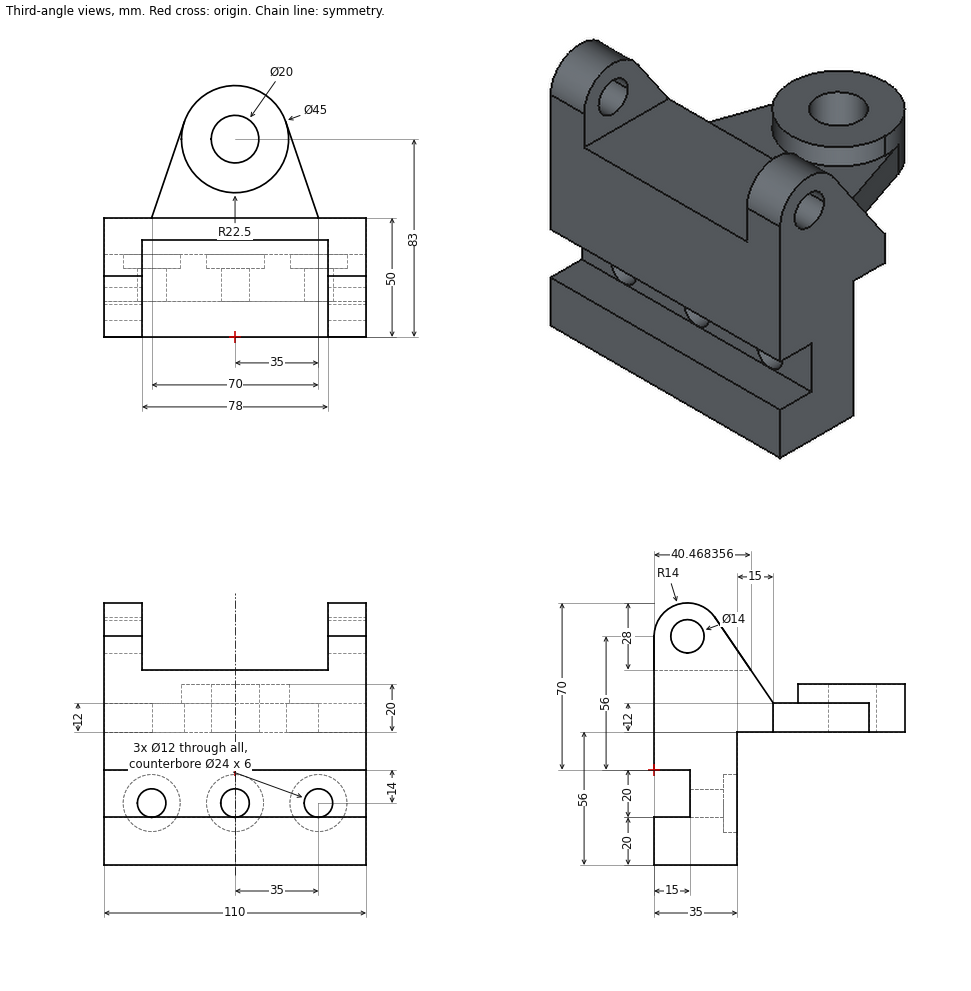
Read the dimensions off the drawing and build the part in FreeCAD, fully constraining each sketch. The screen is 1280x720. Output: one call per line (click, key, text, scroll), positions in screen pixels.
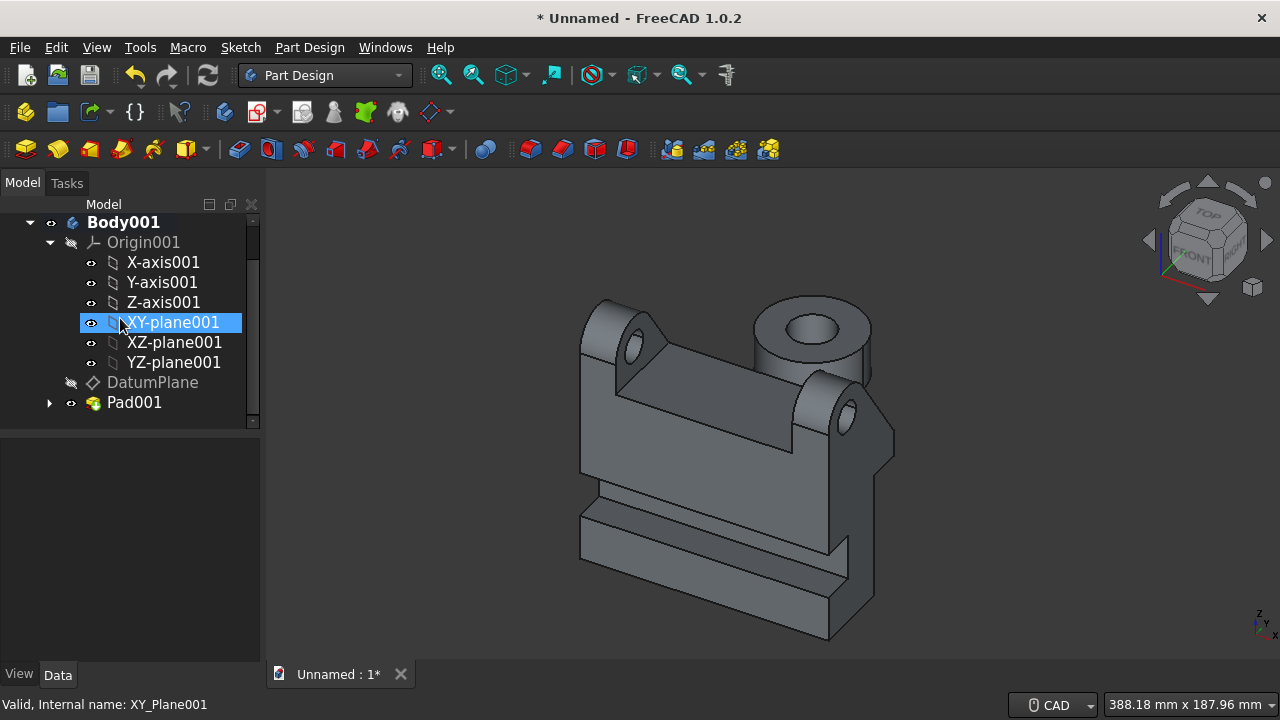
scroll(120, 318, up, 15)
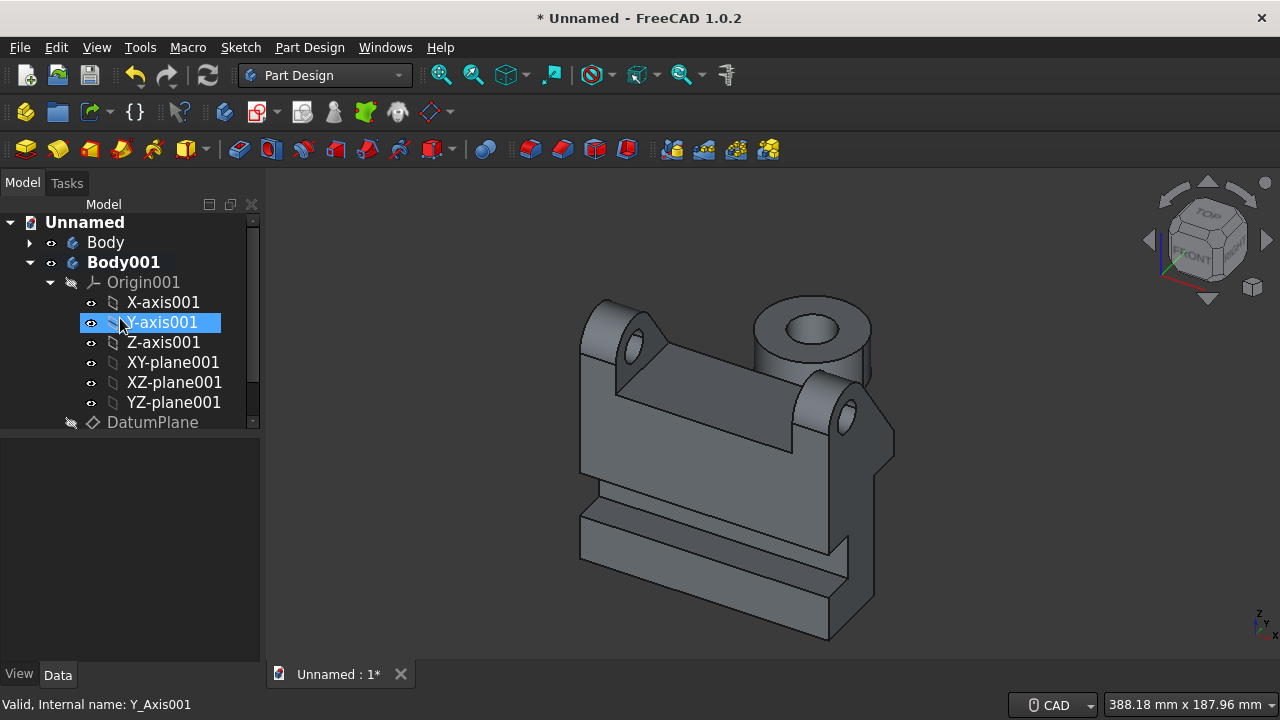
double_click(96, 243)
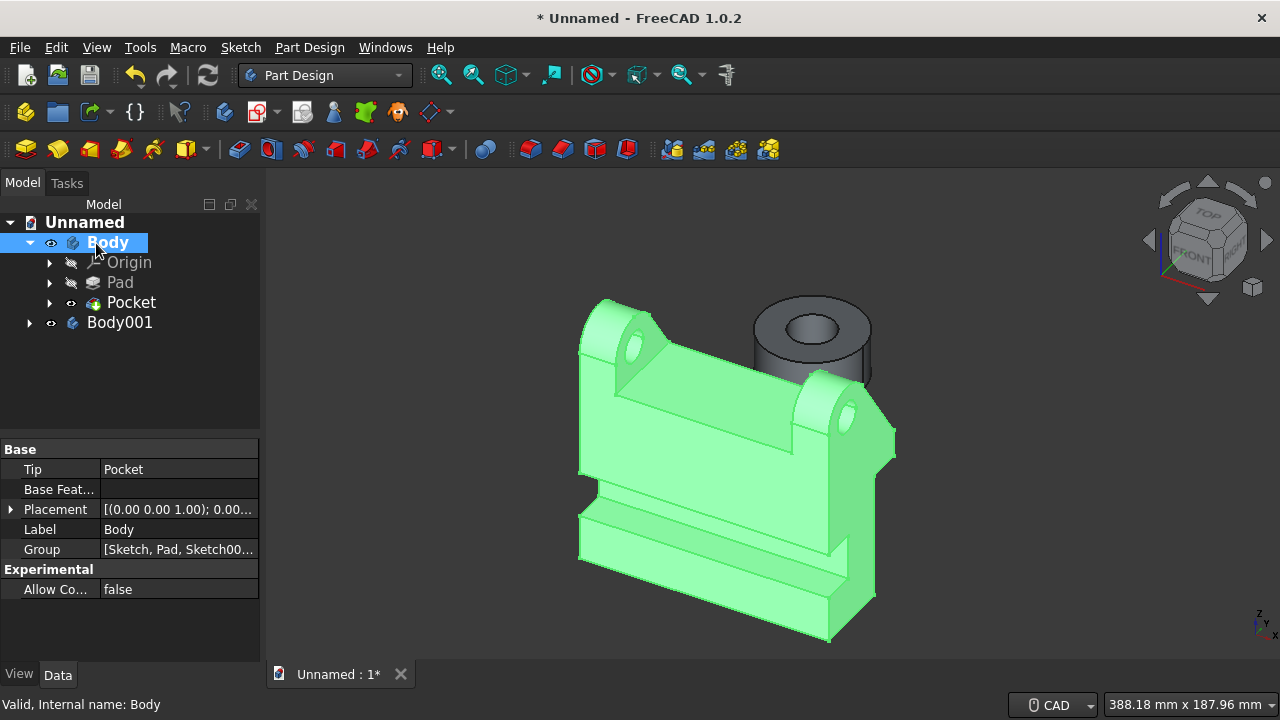
click(96, 243)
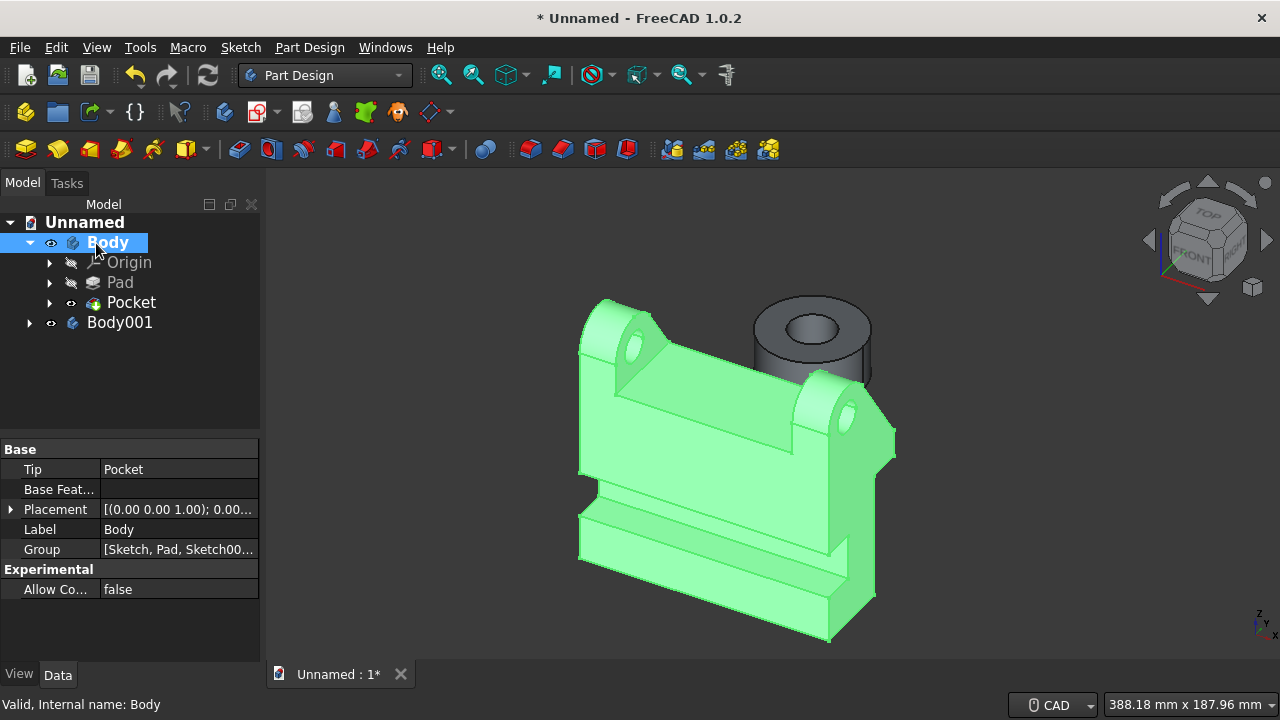
click(146, 589)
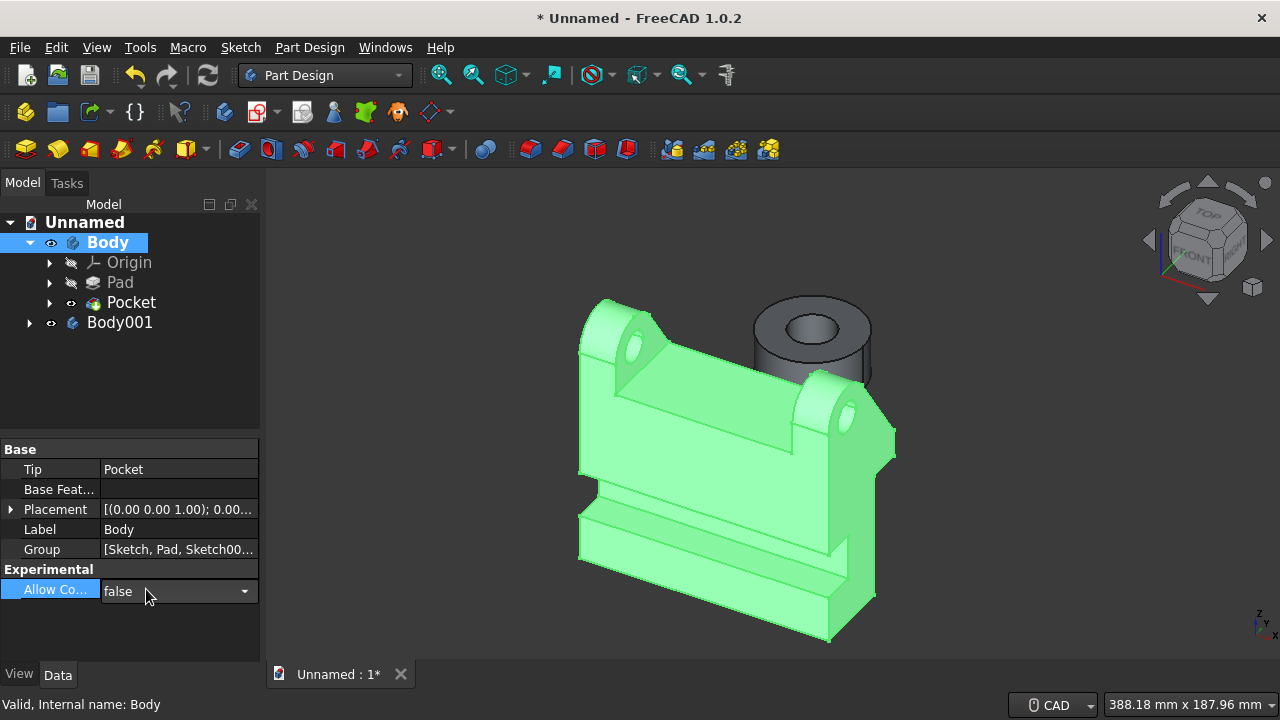
click(146, 589)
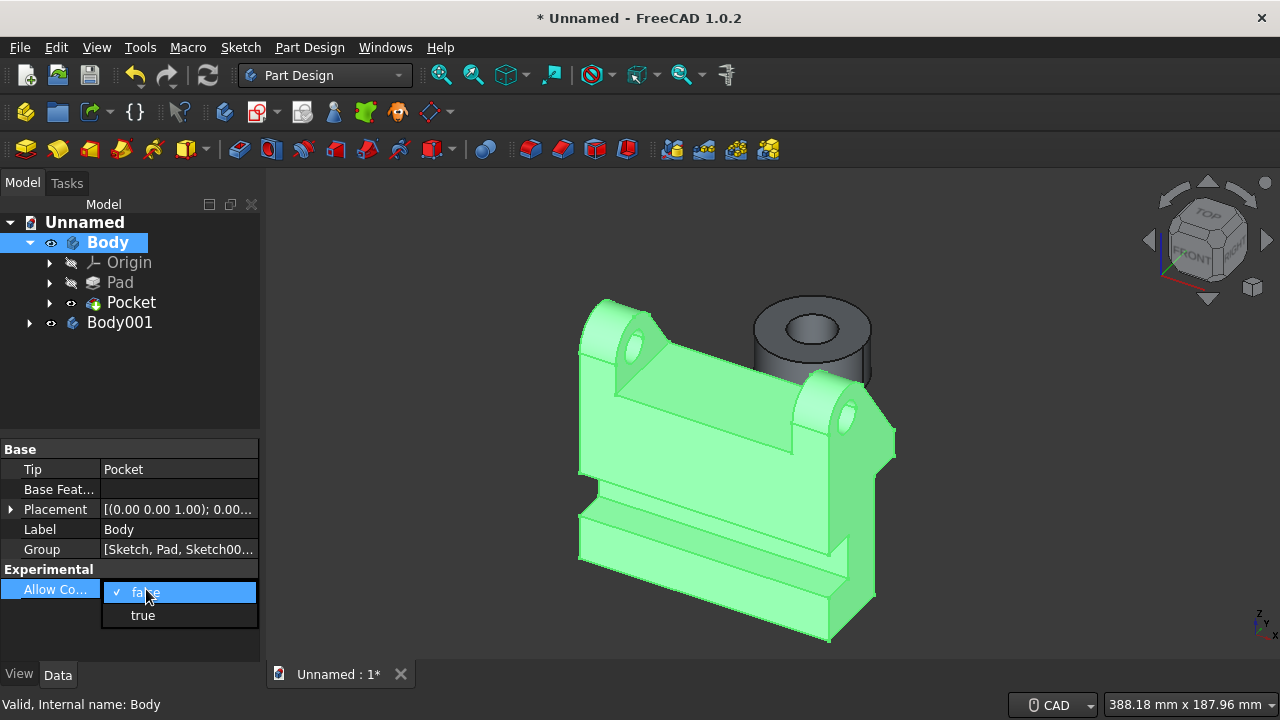
click(179, 616)
key(Return)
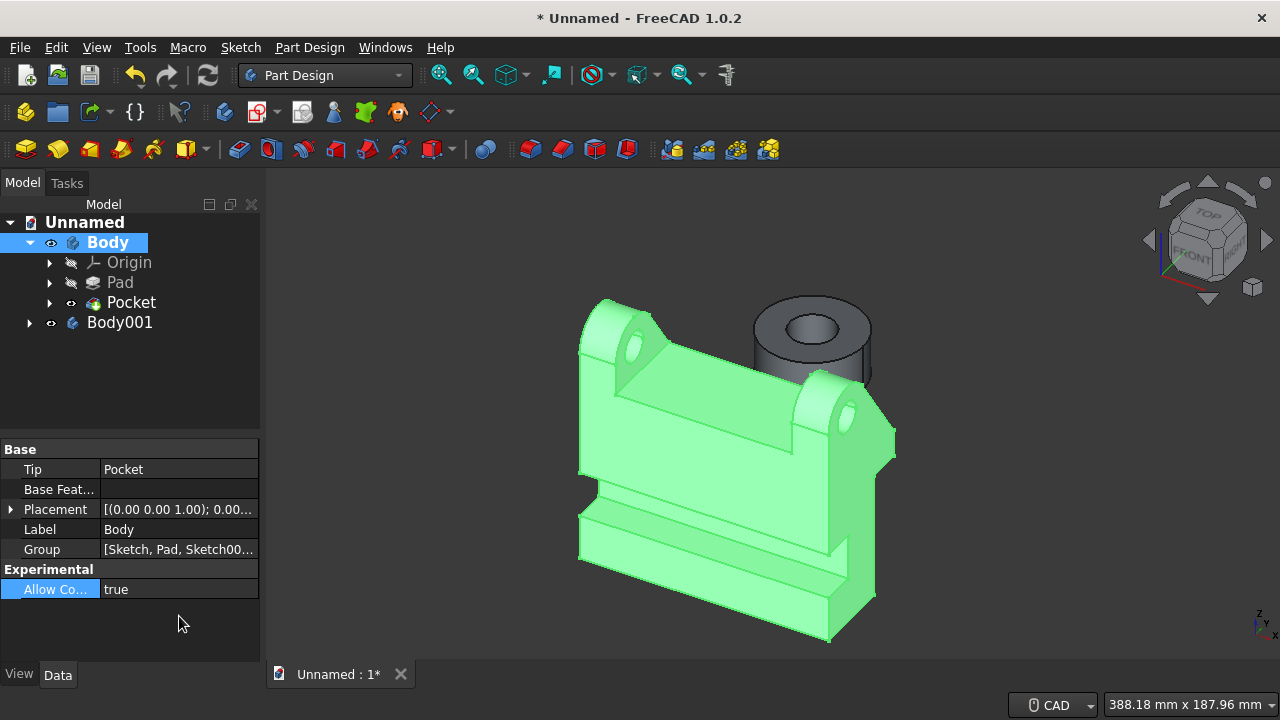
click(96, 323)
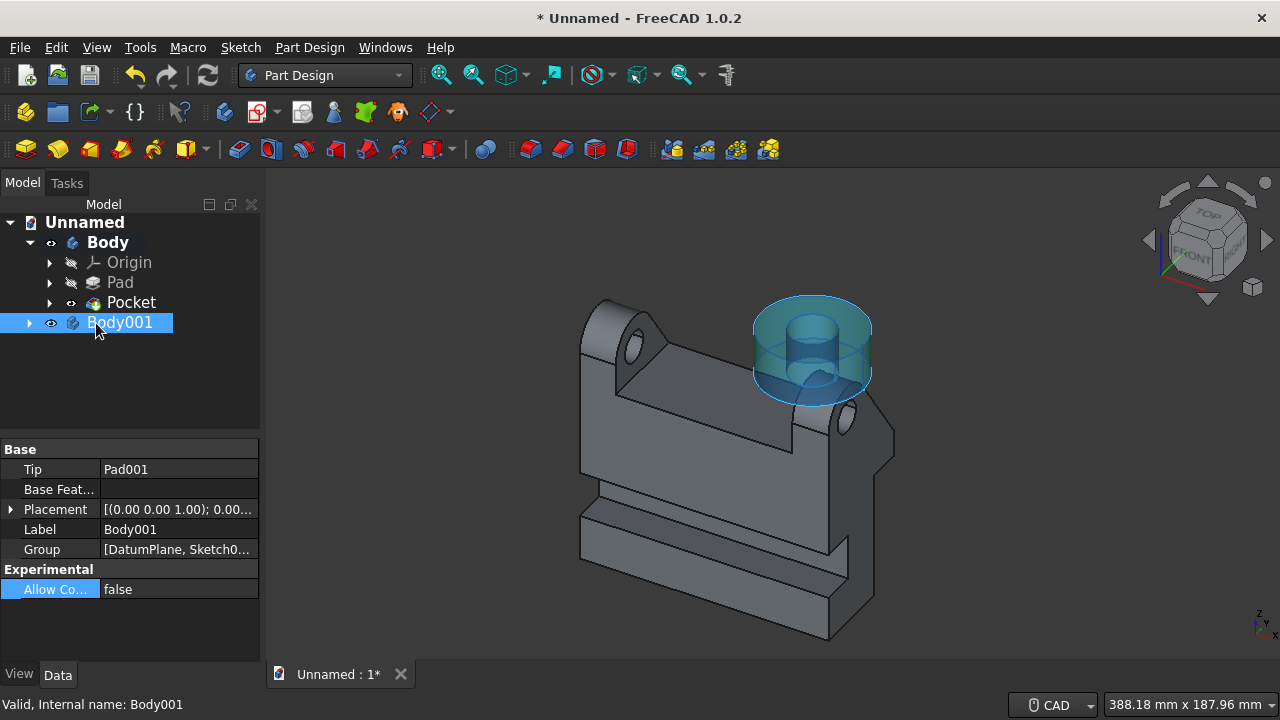
click(486, 150)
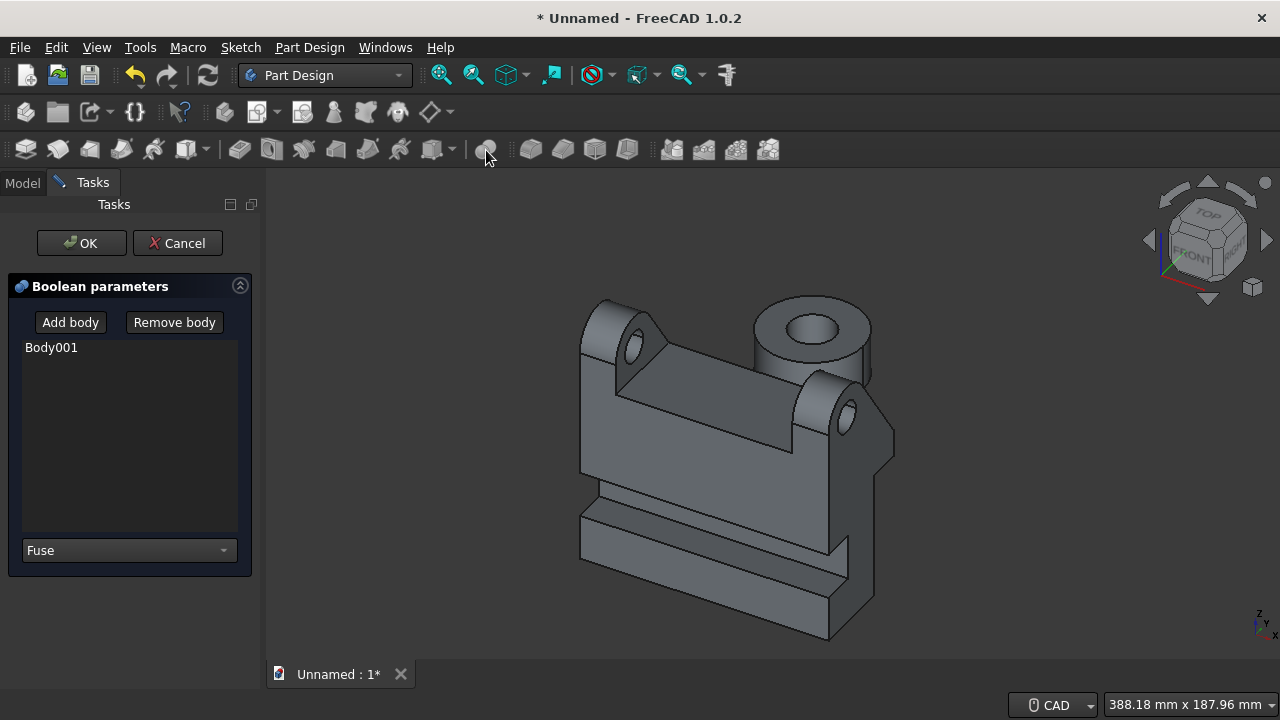
click(82, 243)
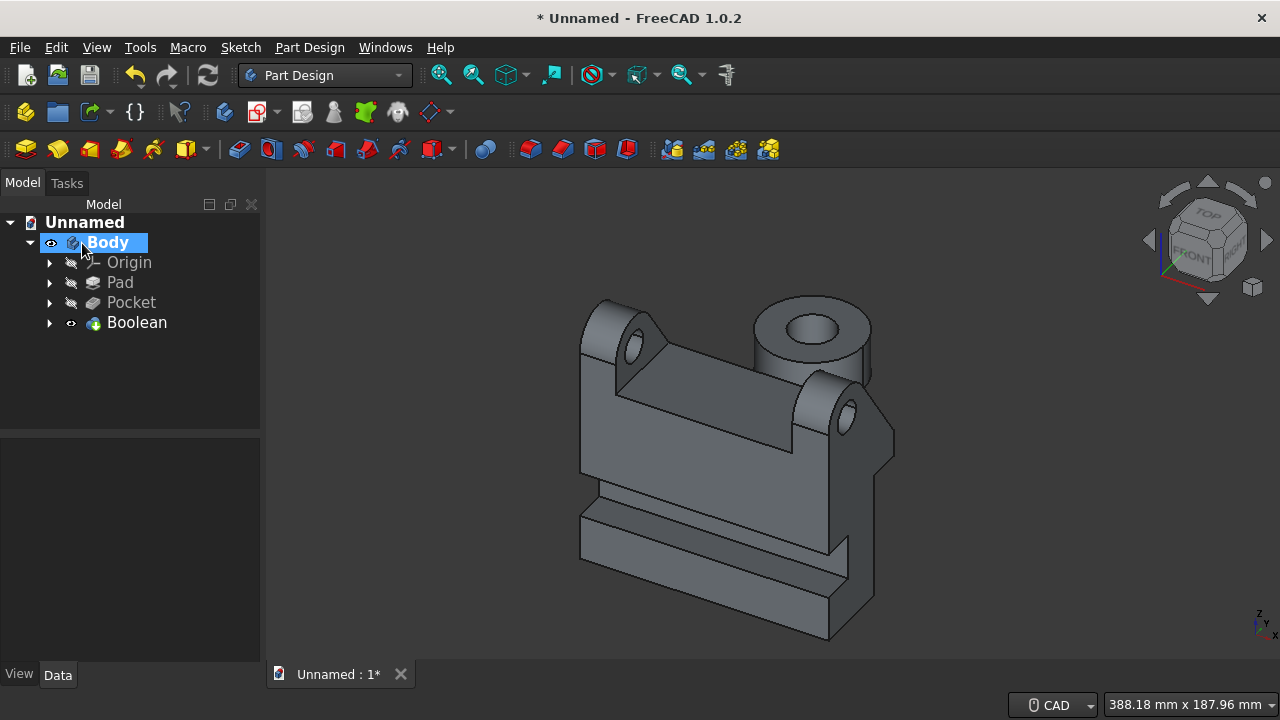
key(5)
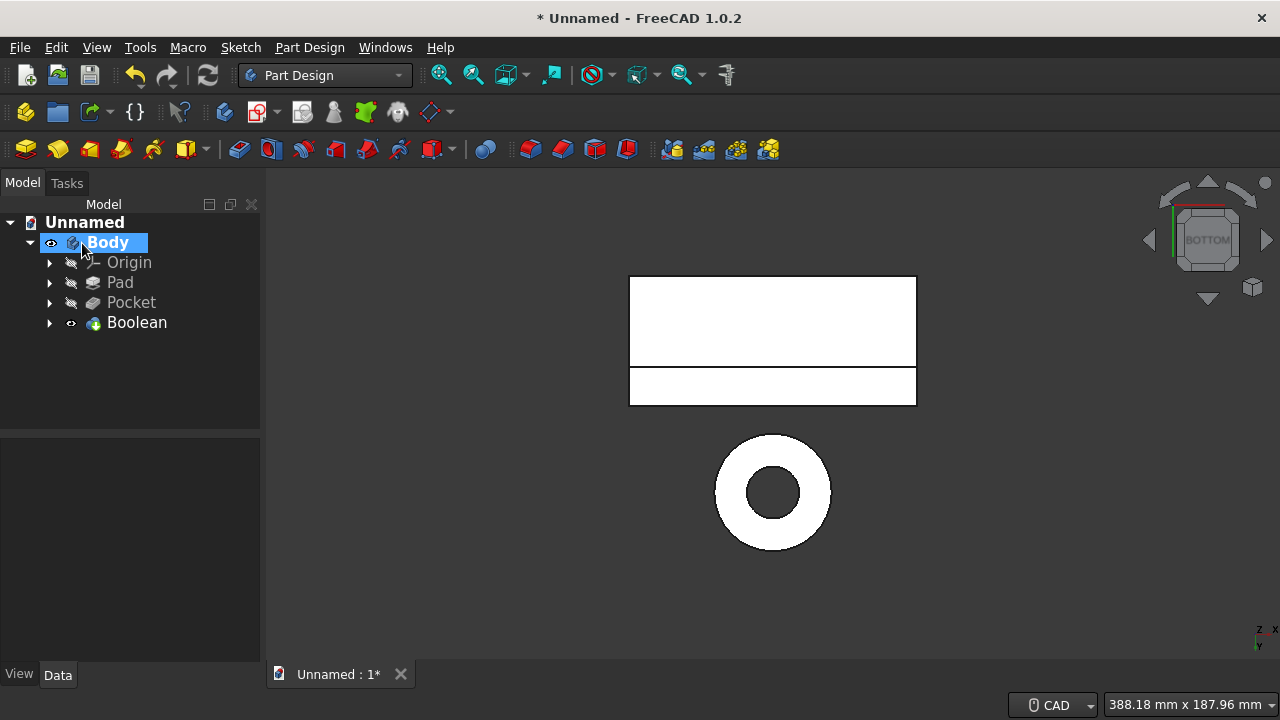
click(855, 386)